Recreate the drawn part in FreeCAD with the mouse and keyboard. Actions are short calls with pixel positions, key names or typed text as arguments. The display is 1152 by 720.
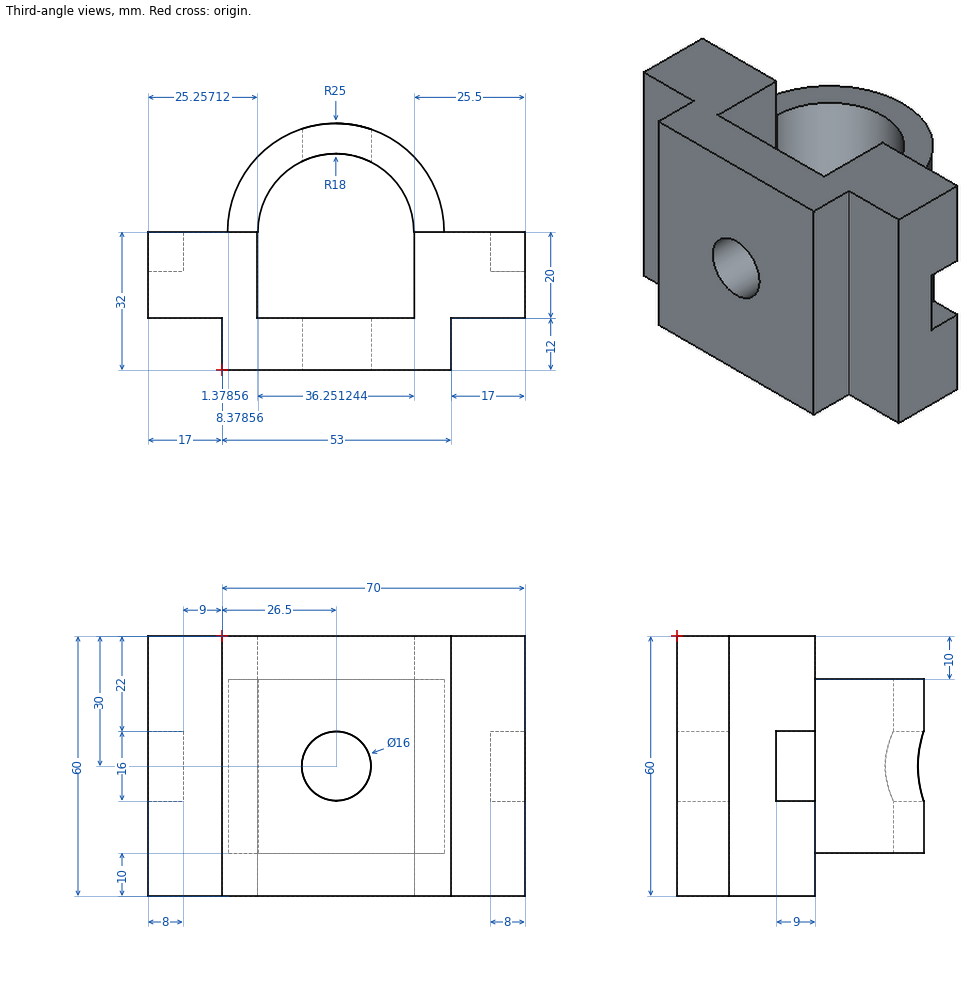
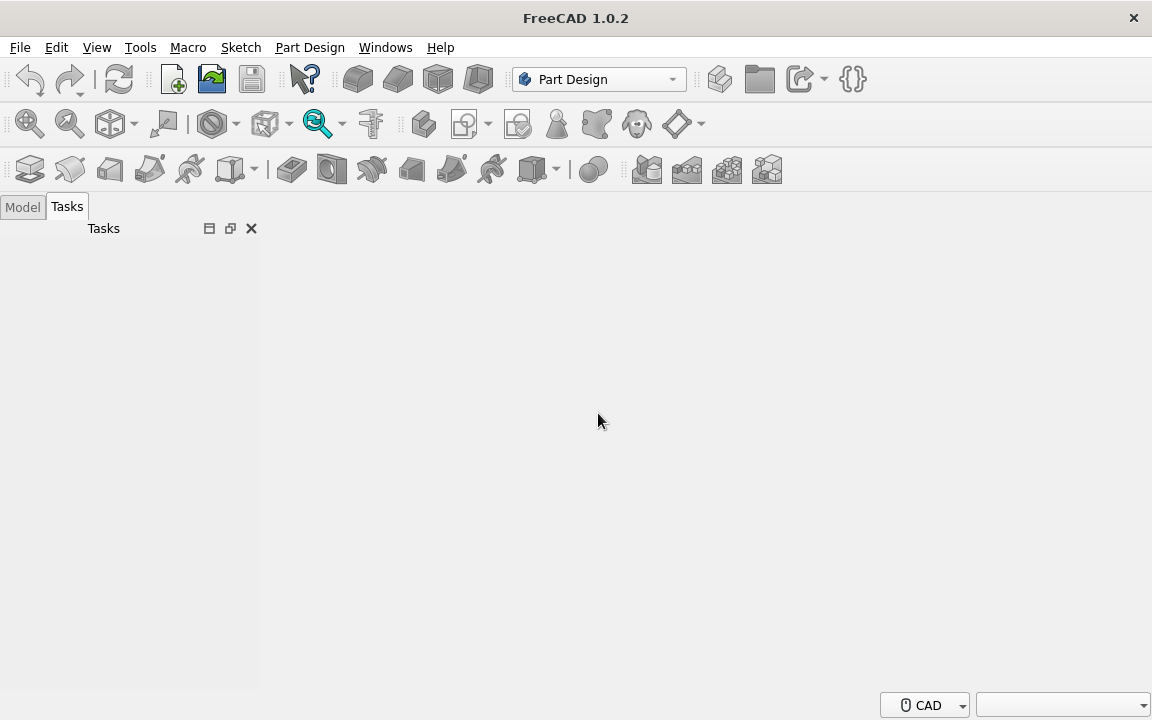
key(ctrl+n)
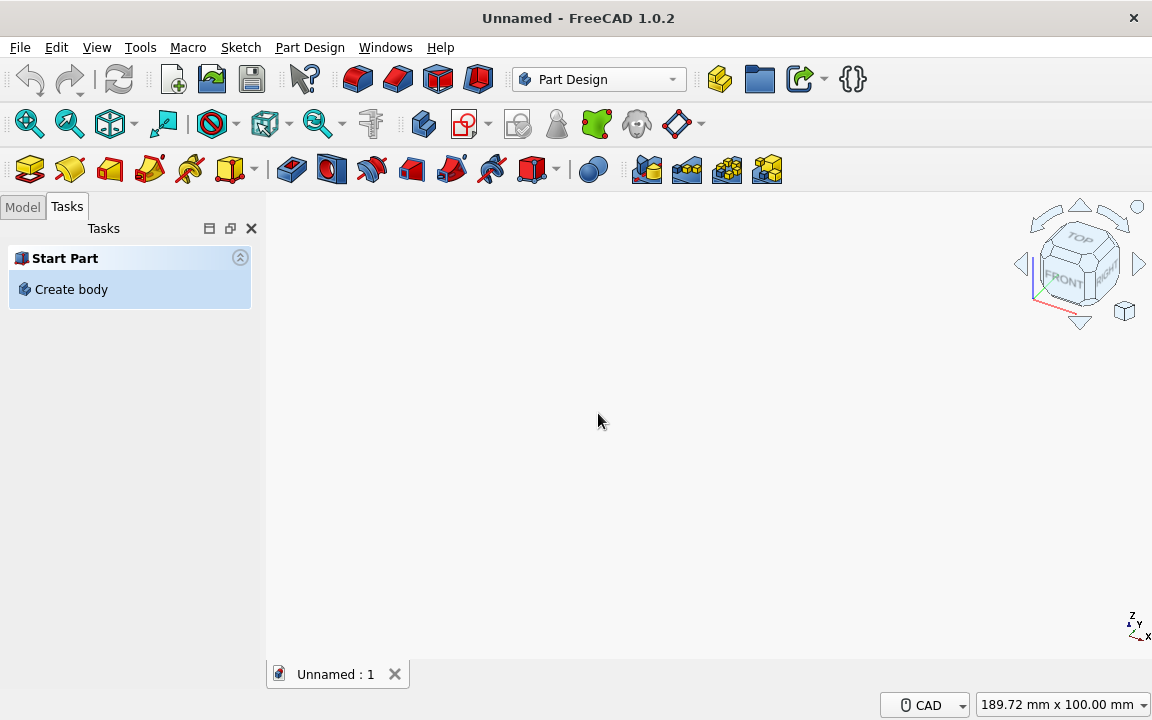
click(464, 124)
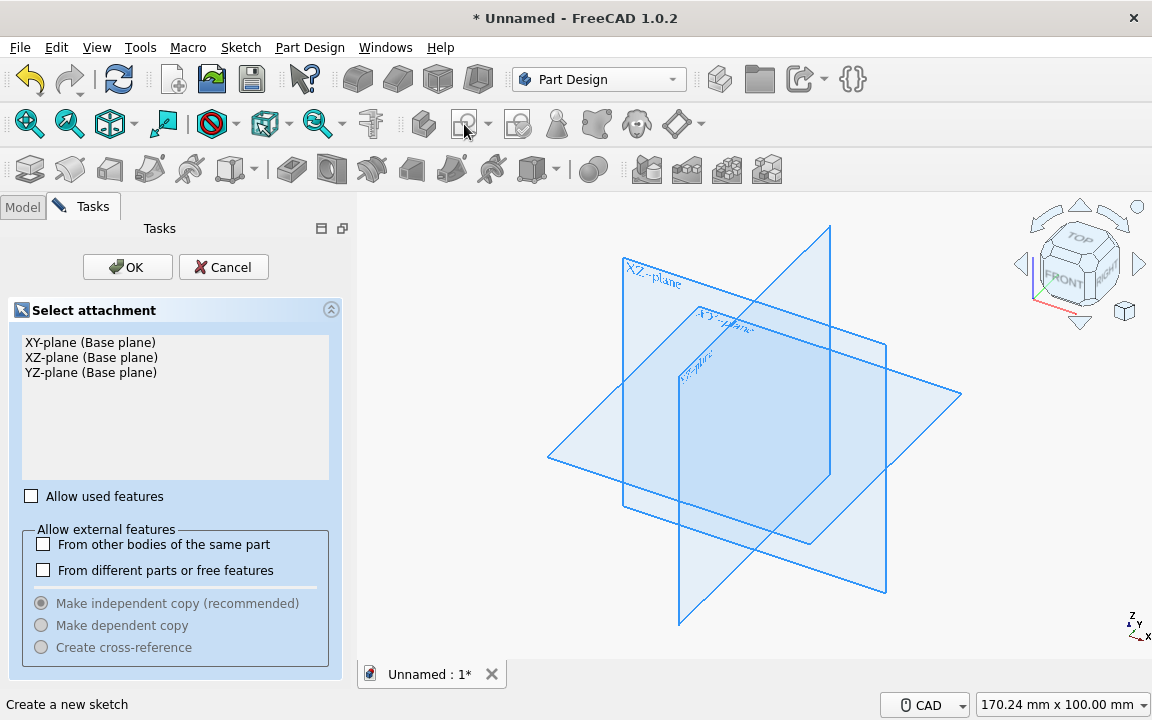
click(82, 342)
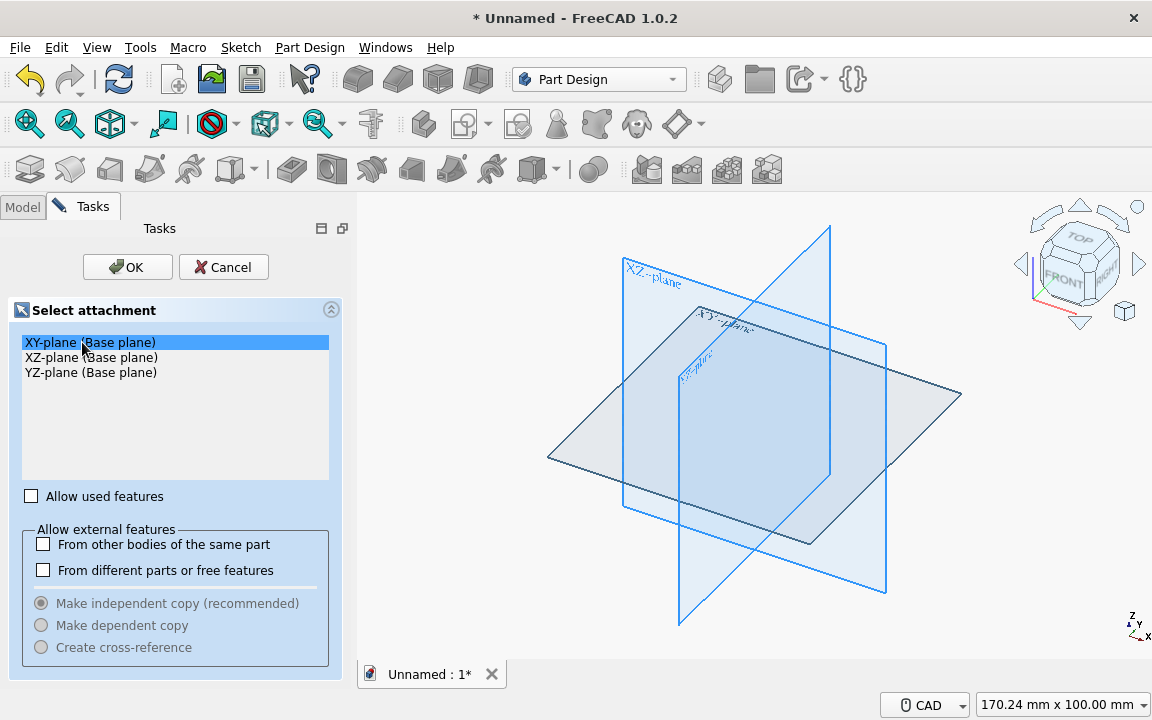
click(128, 267)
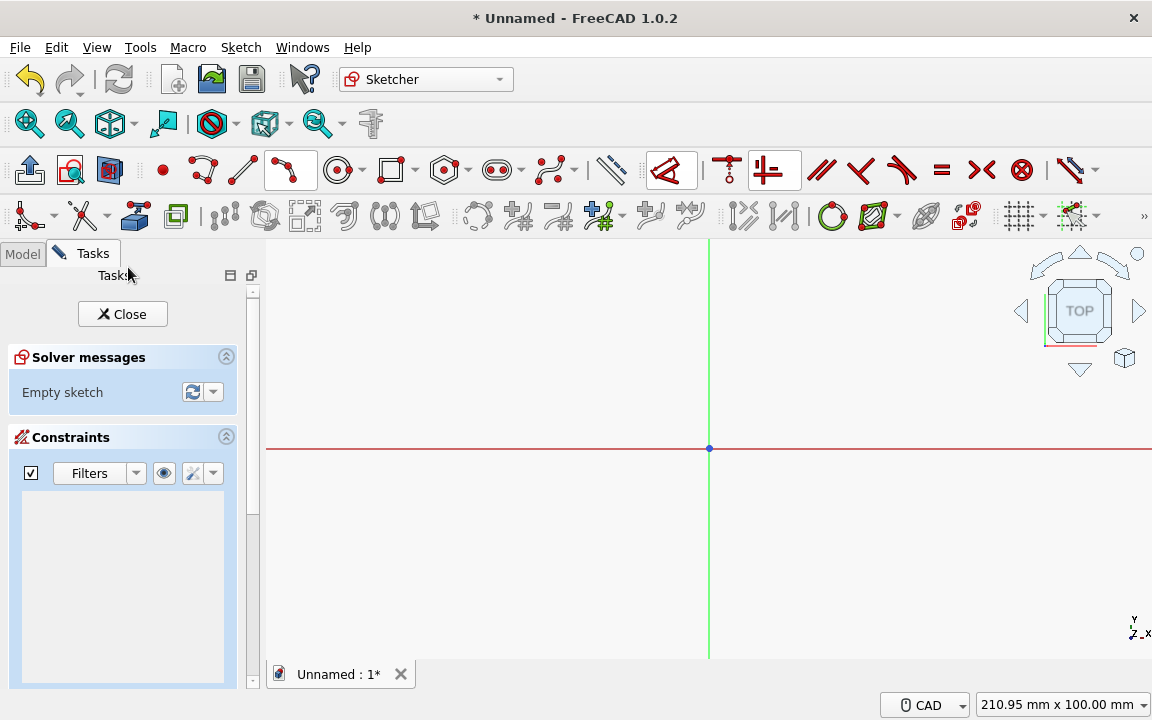
scroll(294, 631, down, 1)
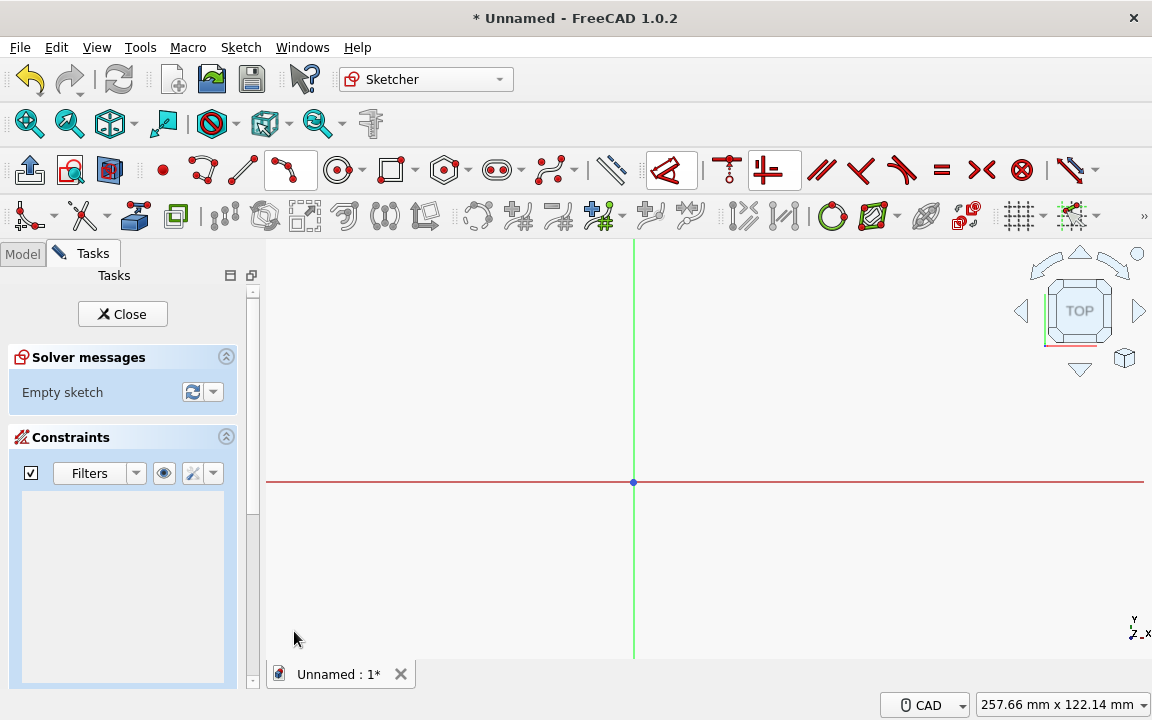
scroll(897, 383, up, 2)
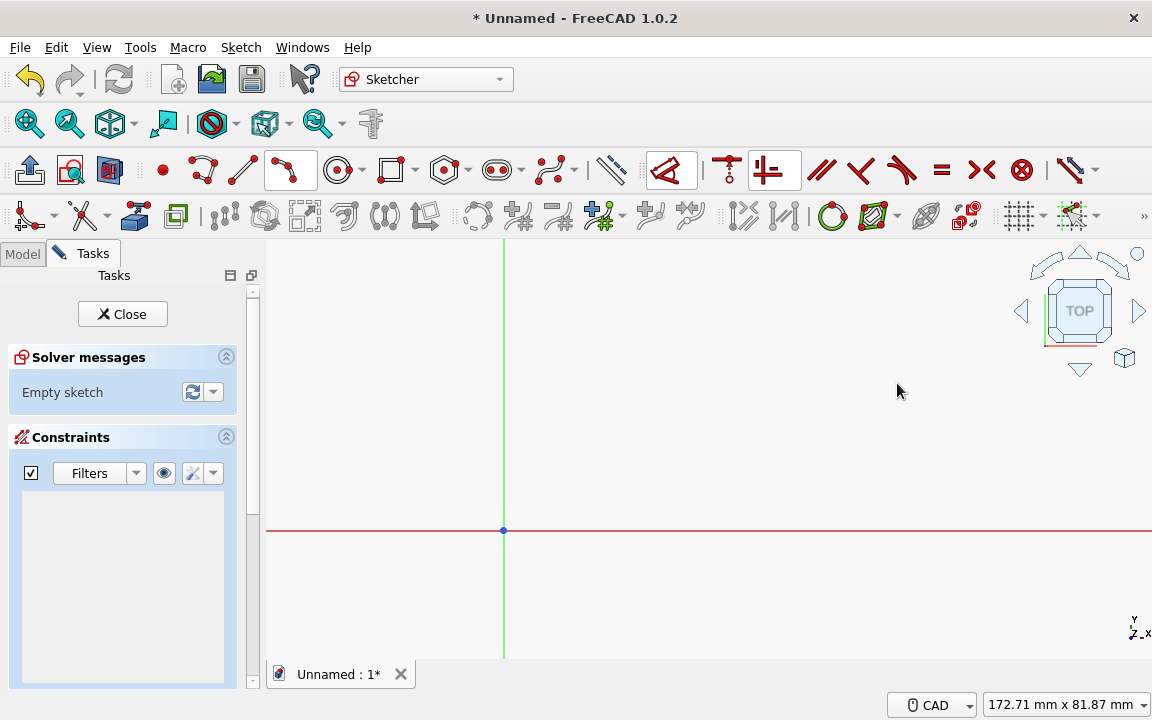
key(g)
key(m)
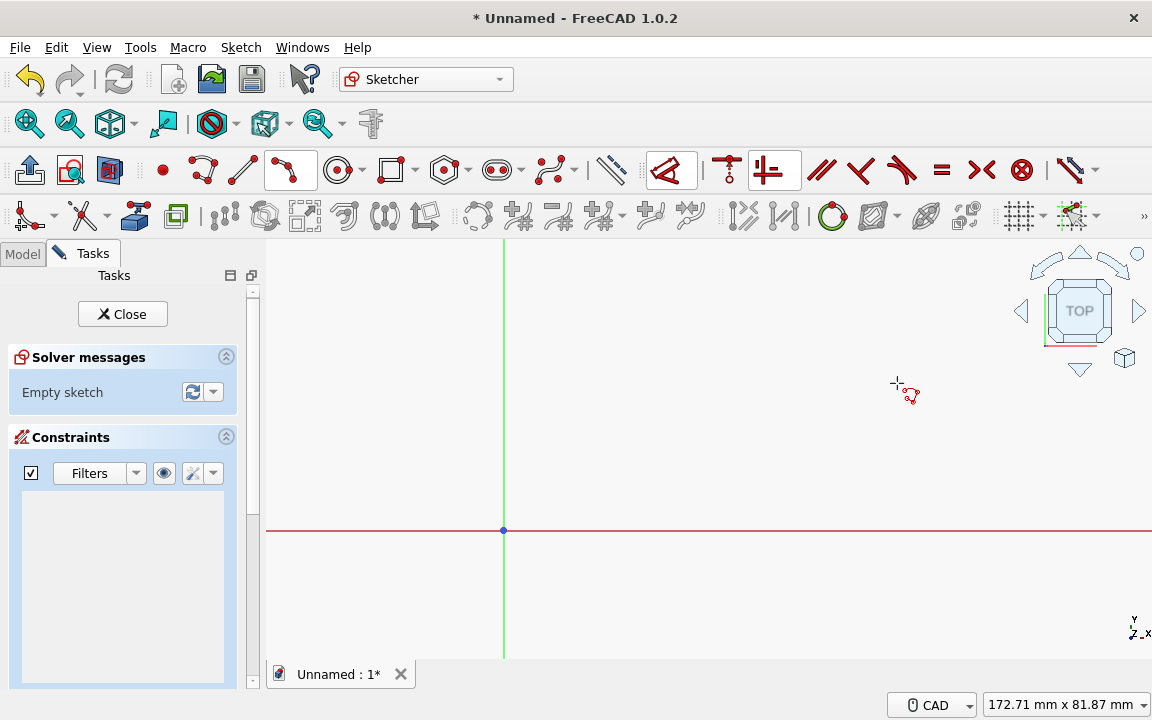
click(504, 531)
click(776, 522)
click(776, 469)
click(863, 469)
click(863, 367)
click(732, 367)
click(738, 469)
click(546, 469)
click(546, 367)
click(417, 367)
click(417, 469)
click(513, 469)
click(504, 531)
key(Escape)
key(Escape)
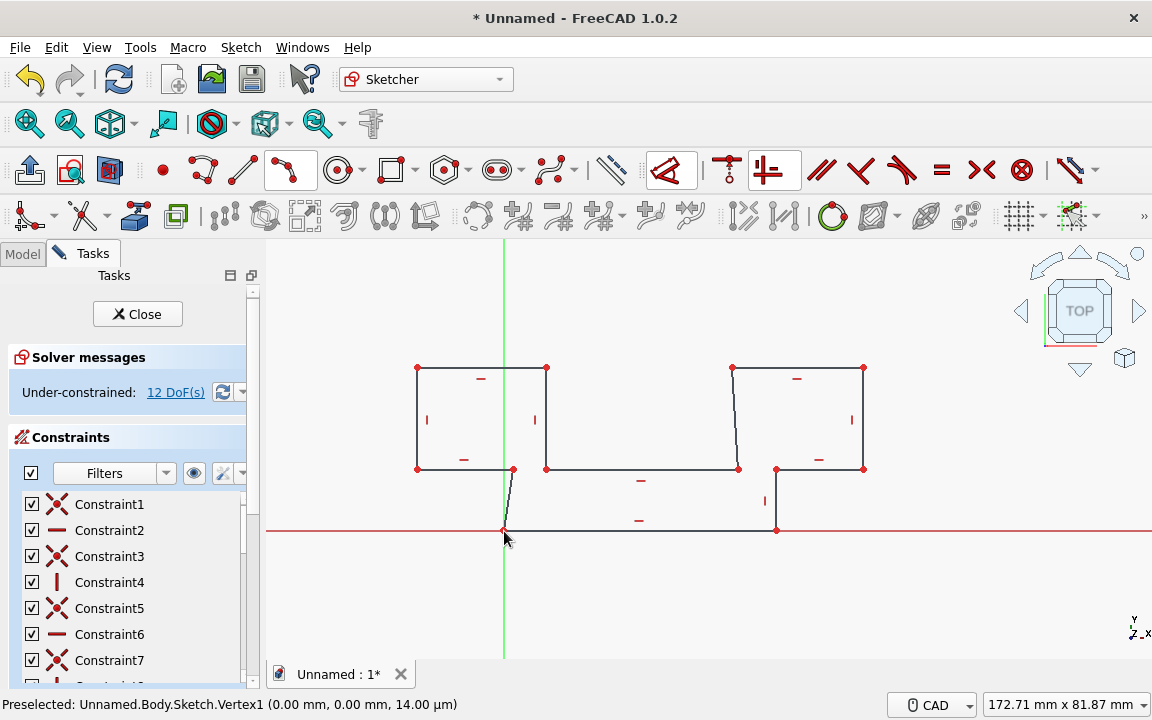
click(507, 513)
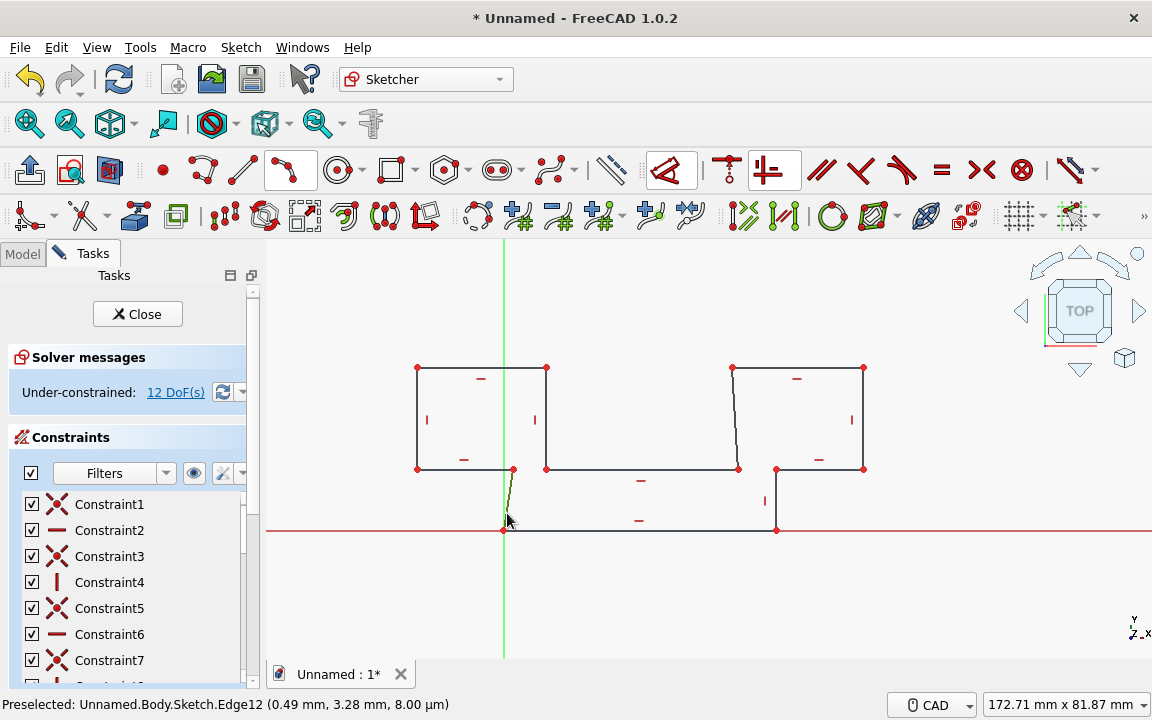
key(v)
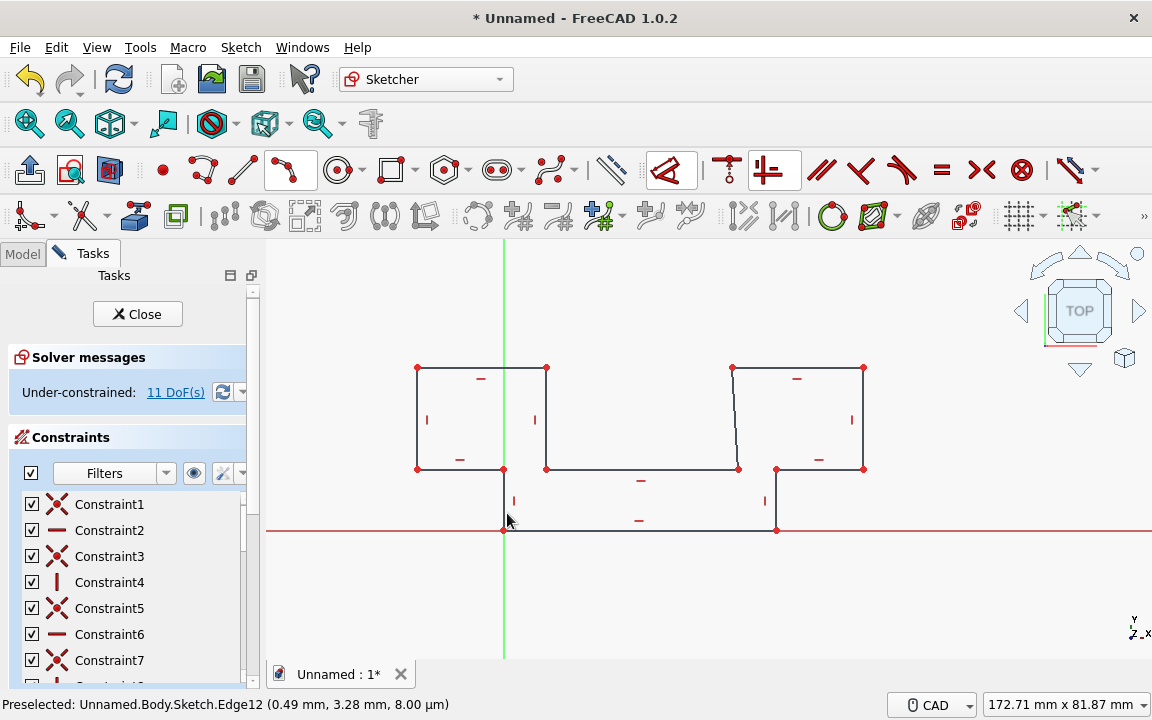
click(586, 531)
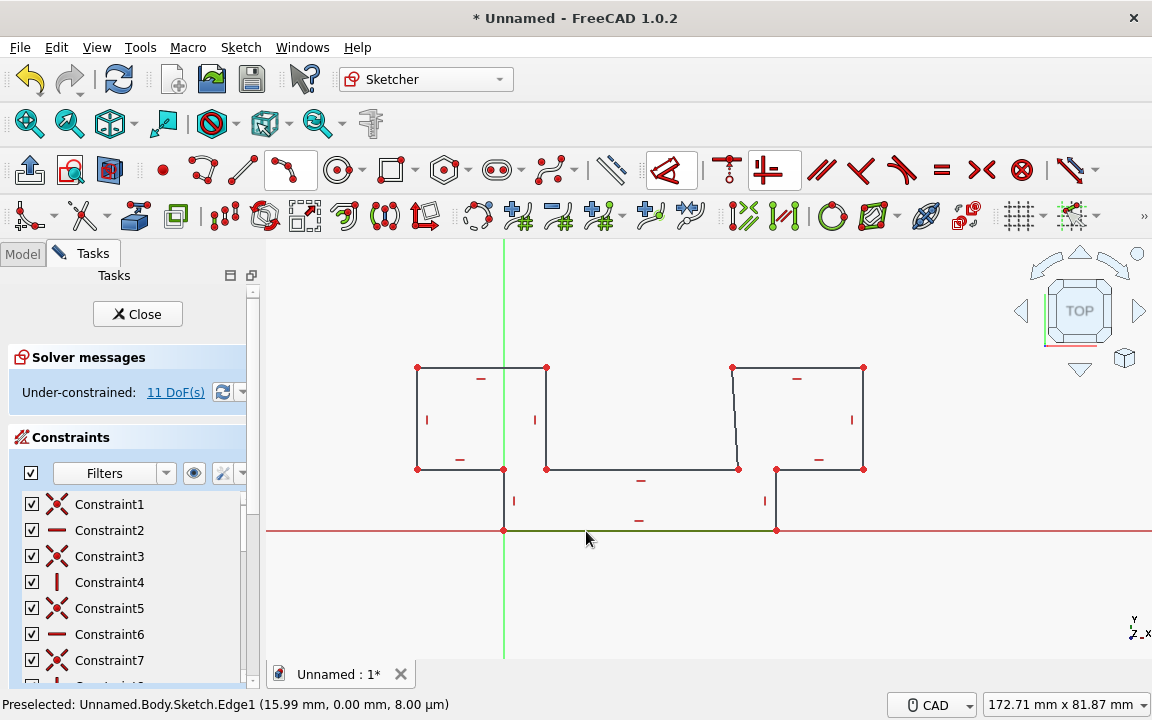
key(l)